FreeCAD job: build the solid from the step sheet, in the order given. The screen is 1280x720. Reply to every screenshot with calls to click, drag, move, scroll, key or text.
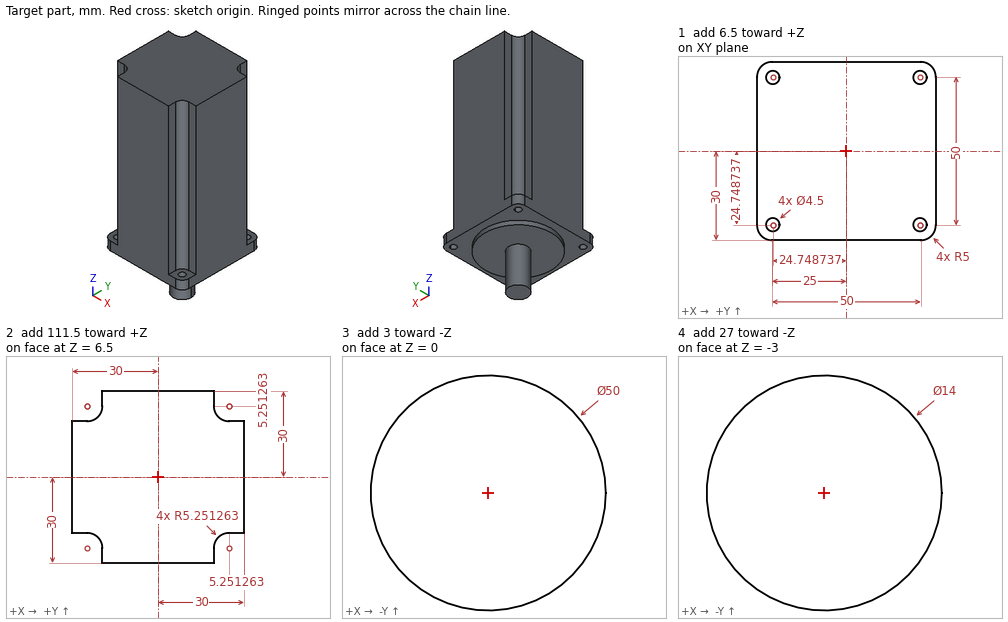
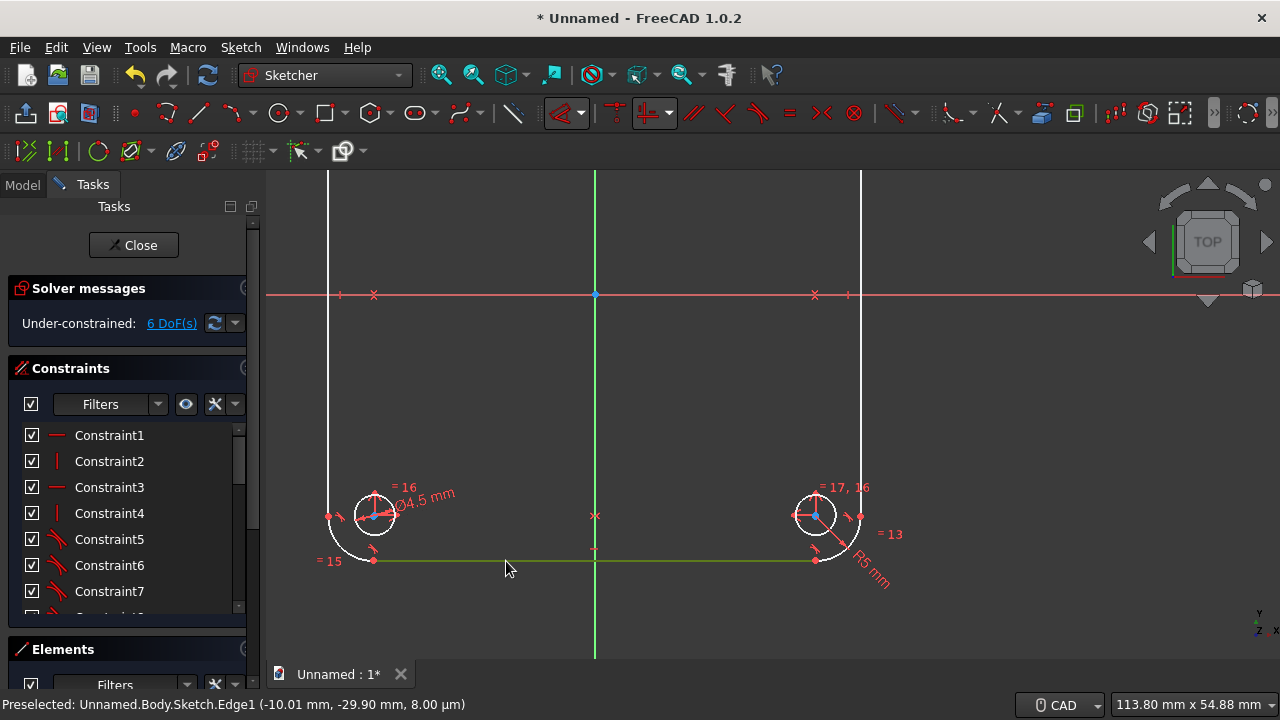
key(l)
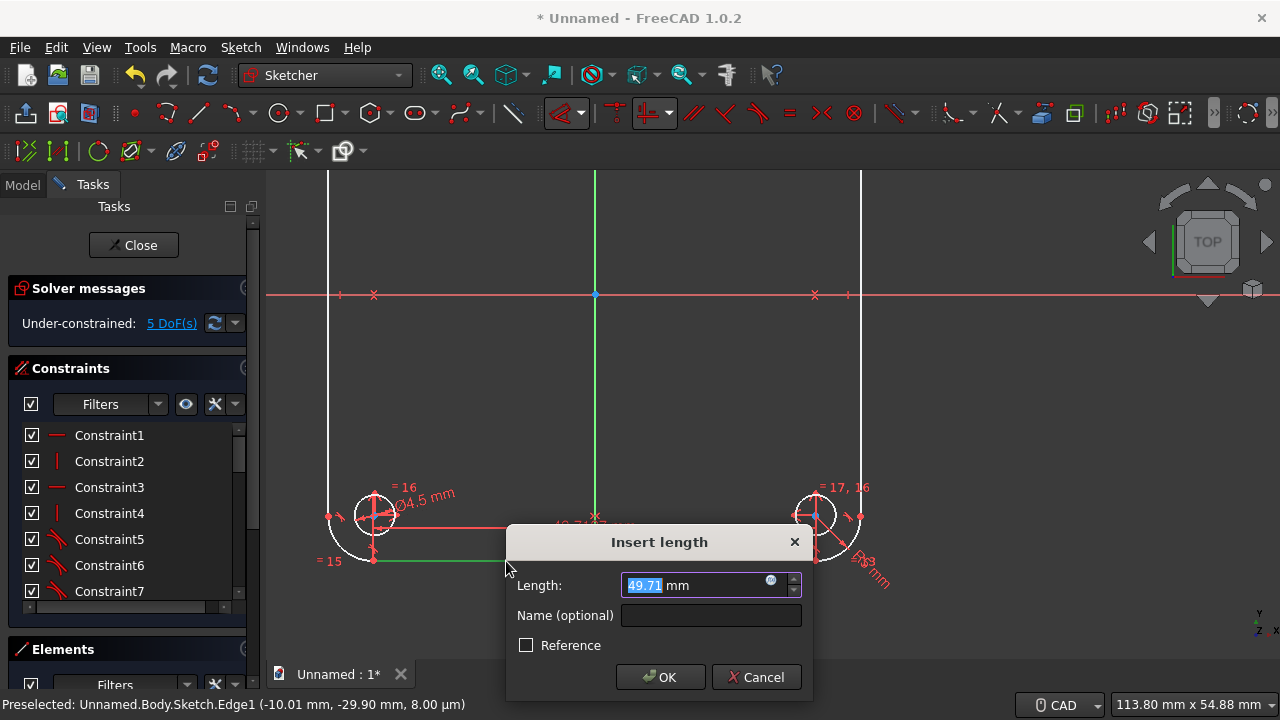
text(50)
key(Return)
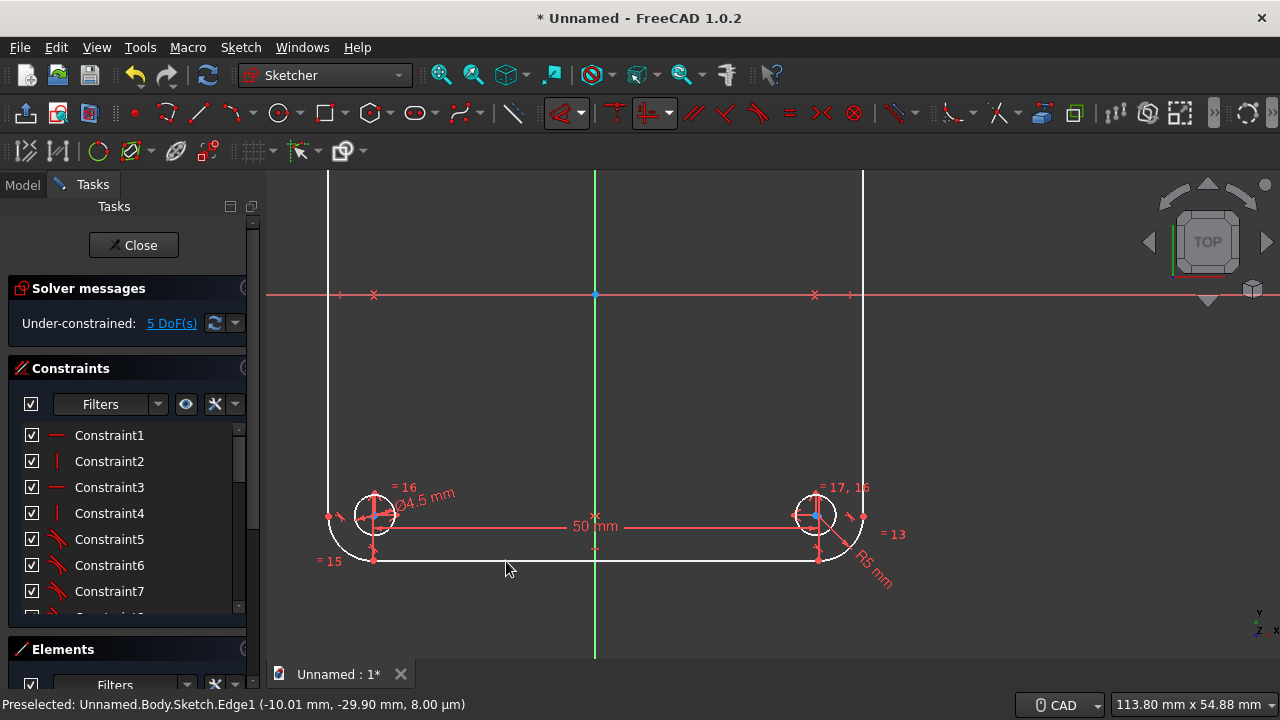
click(863, 383)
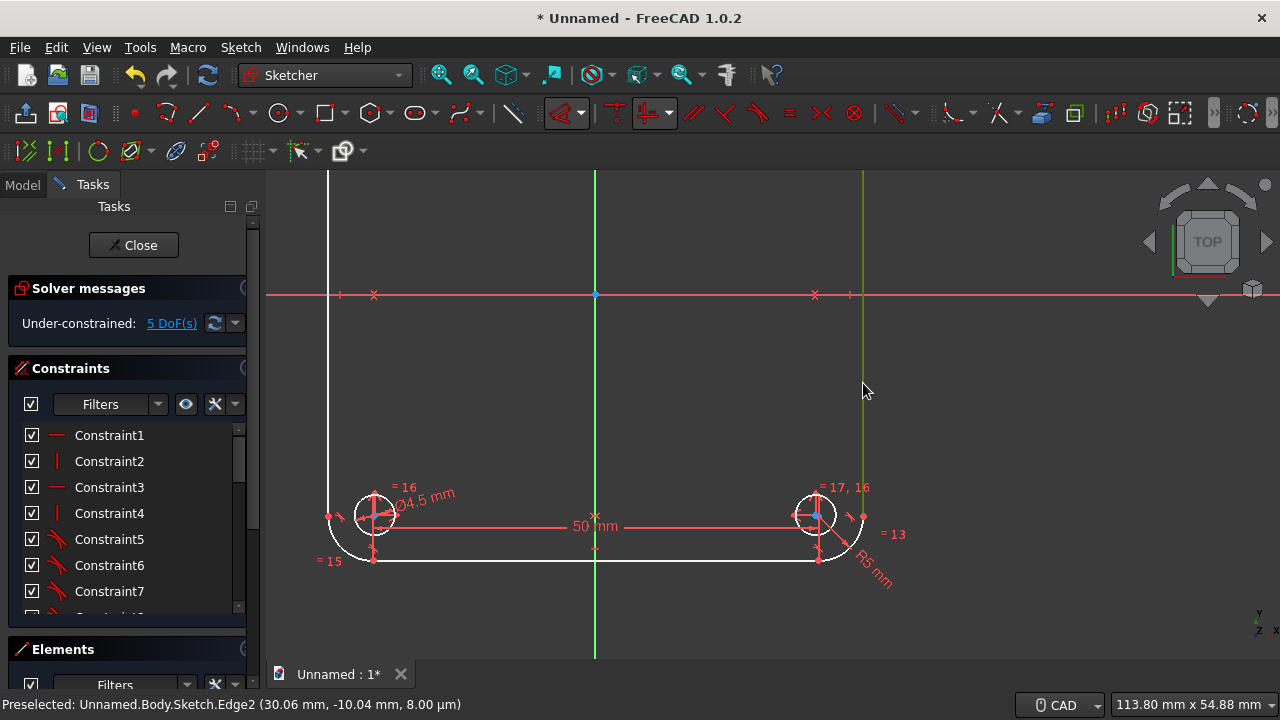
key(i)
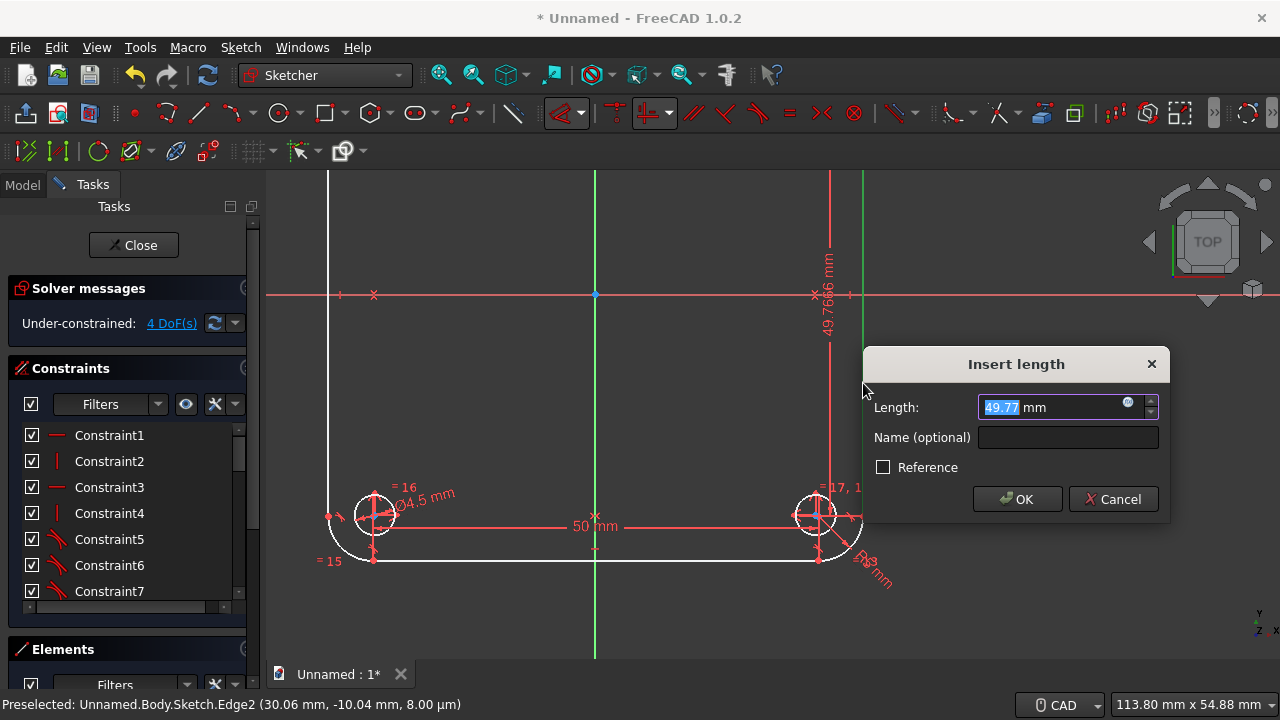
text(50)
key(Return)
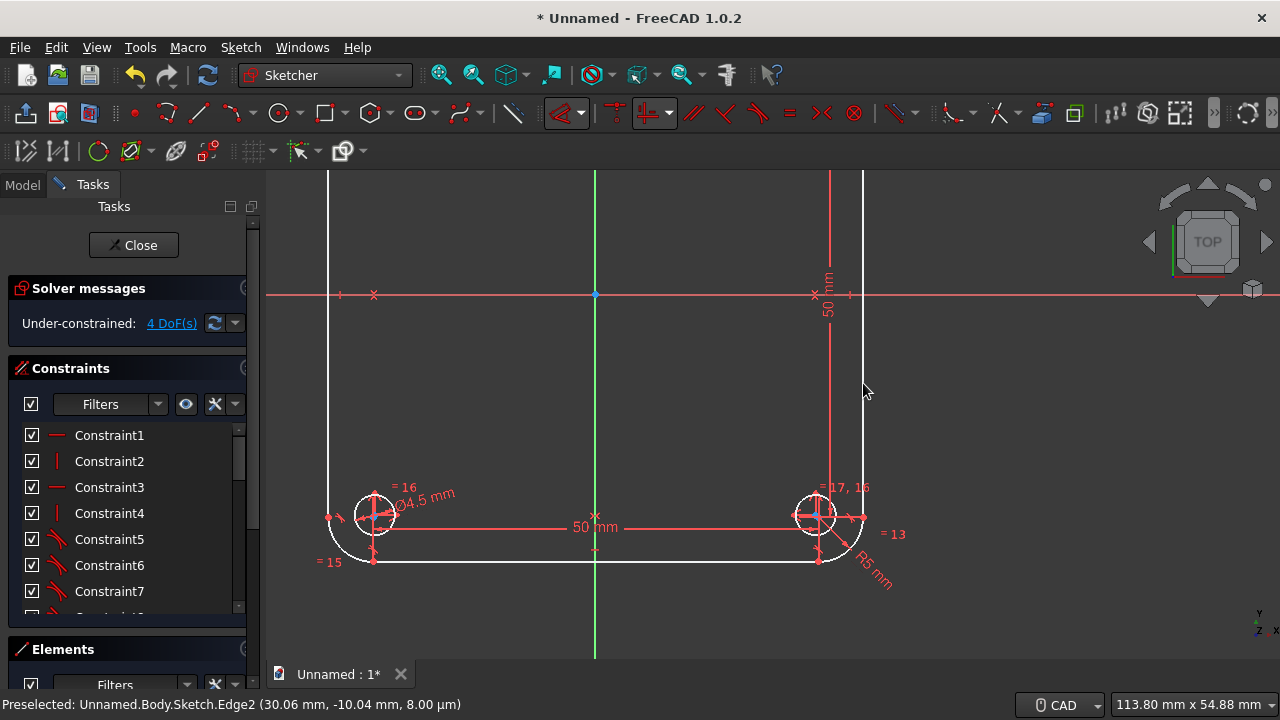
click(373, 562)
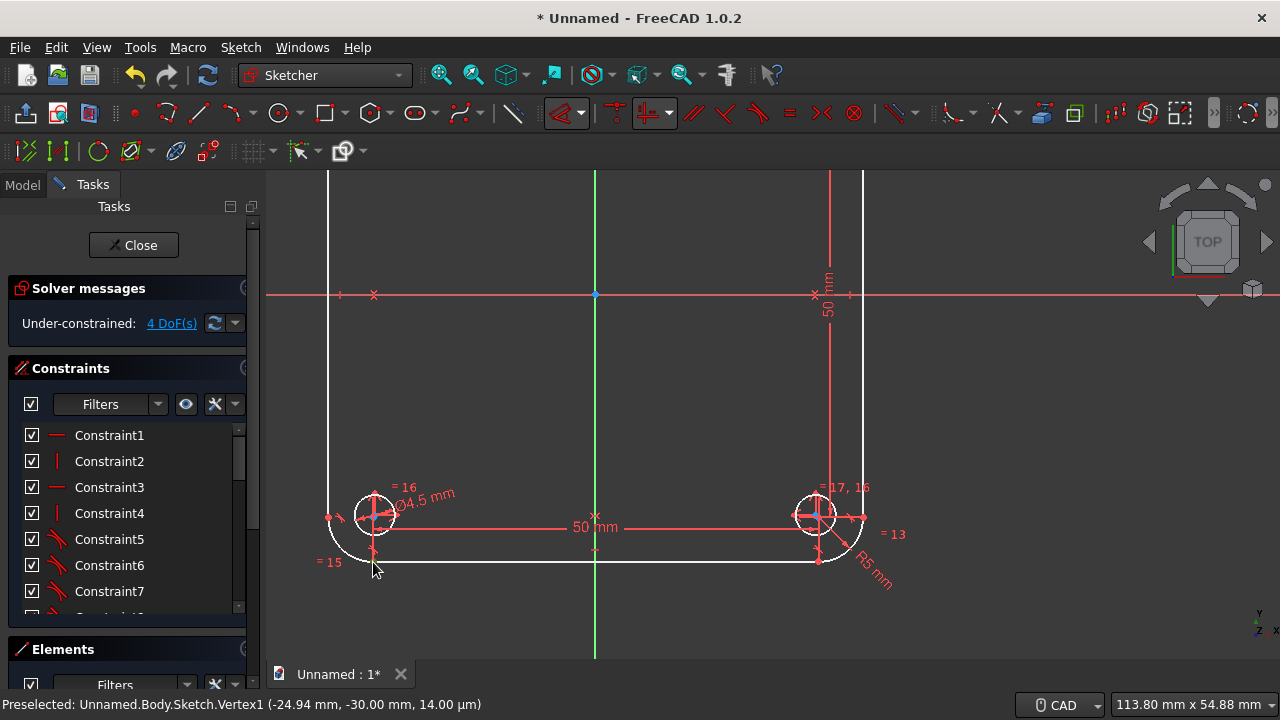
key(l)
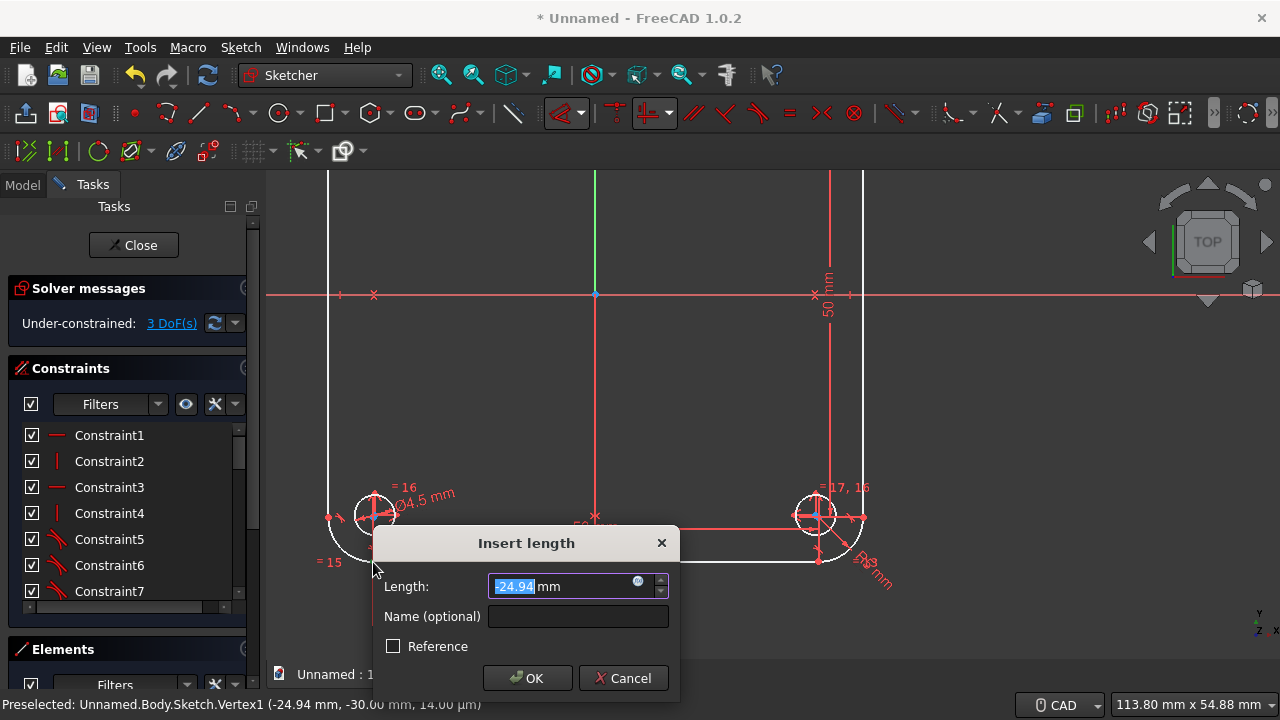
text(-25)
key(Return)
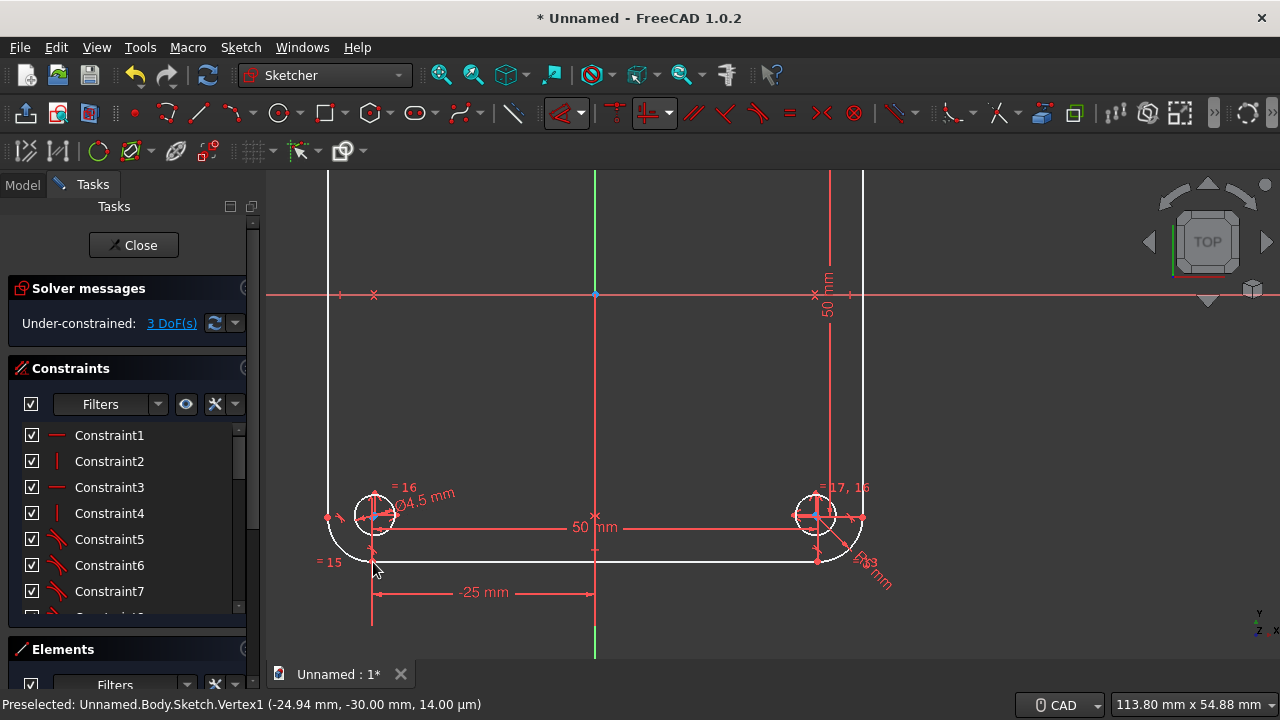
click(372, 562)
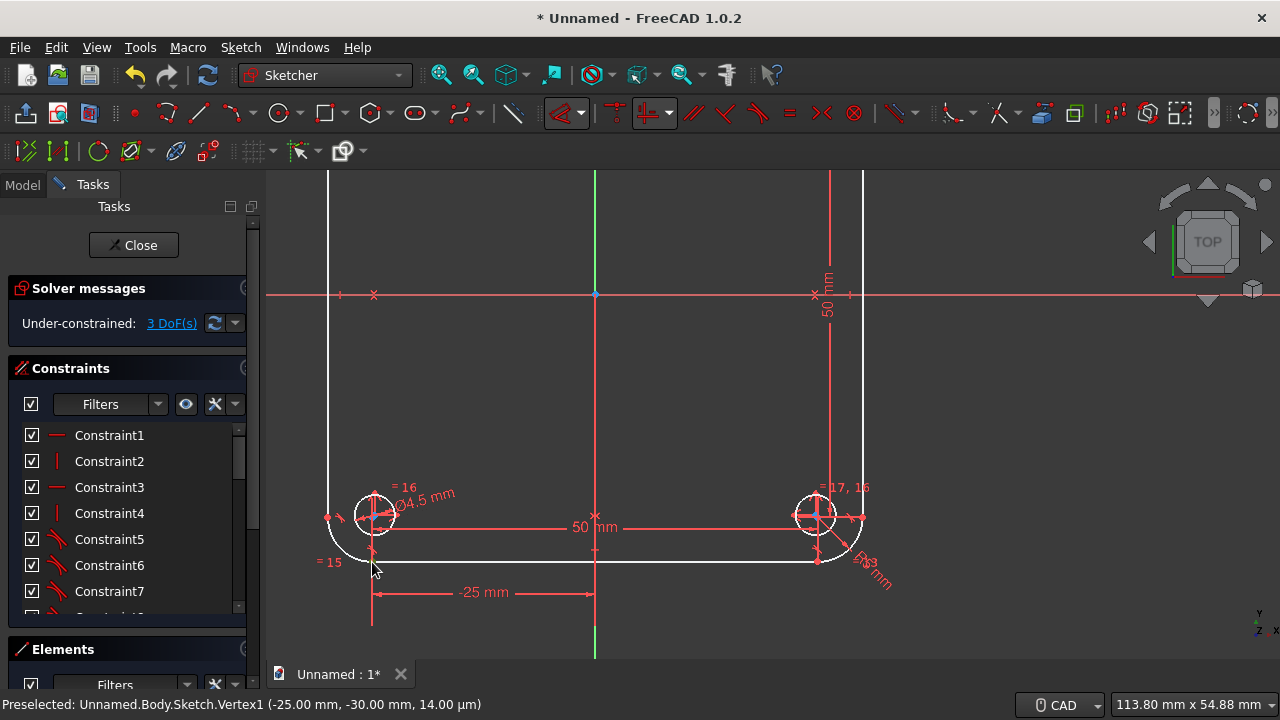
key(i)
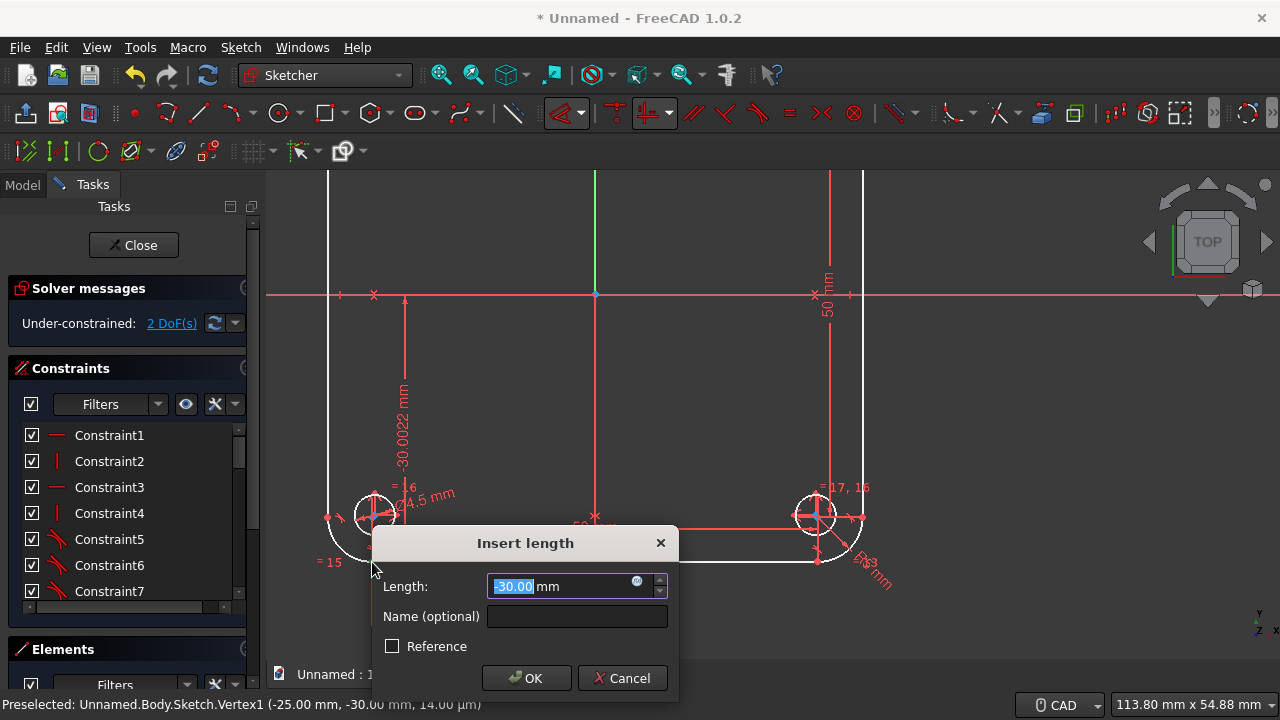
text(-30)
key(Return)